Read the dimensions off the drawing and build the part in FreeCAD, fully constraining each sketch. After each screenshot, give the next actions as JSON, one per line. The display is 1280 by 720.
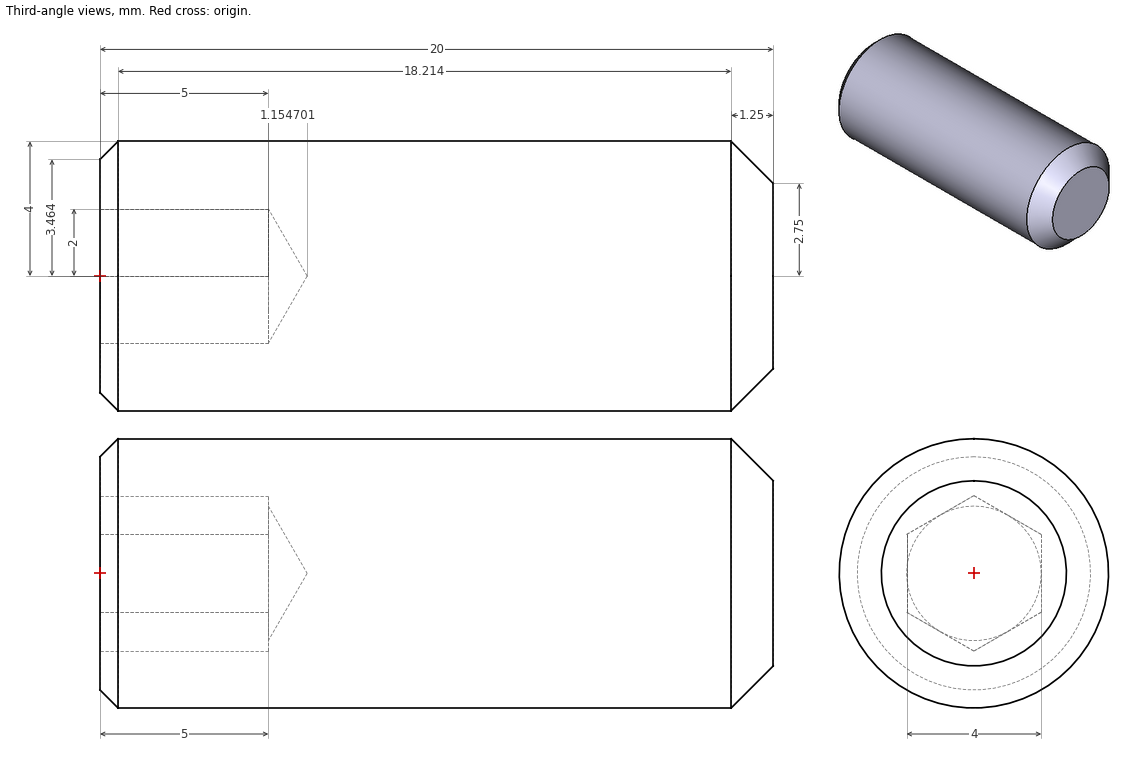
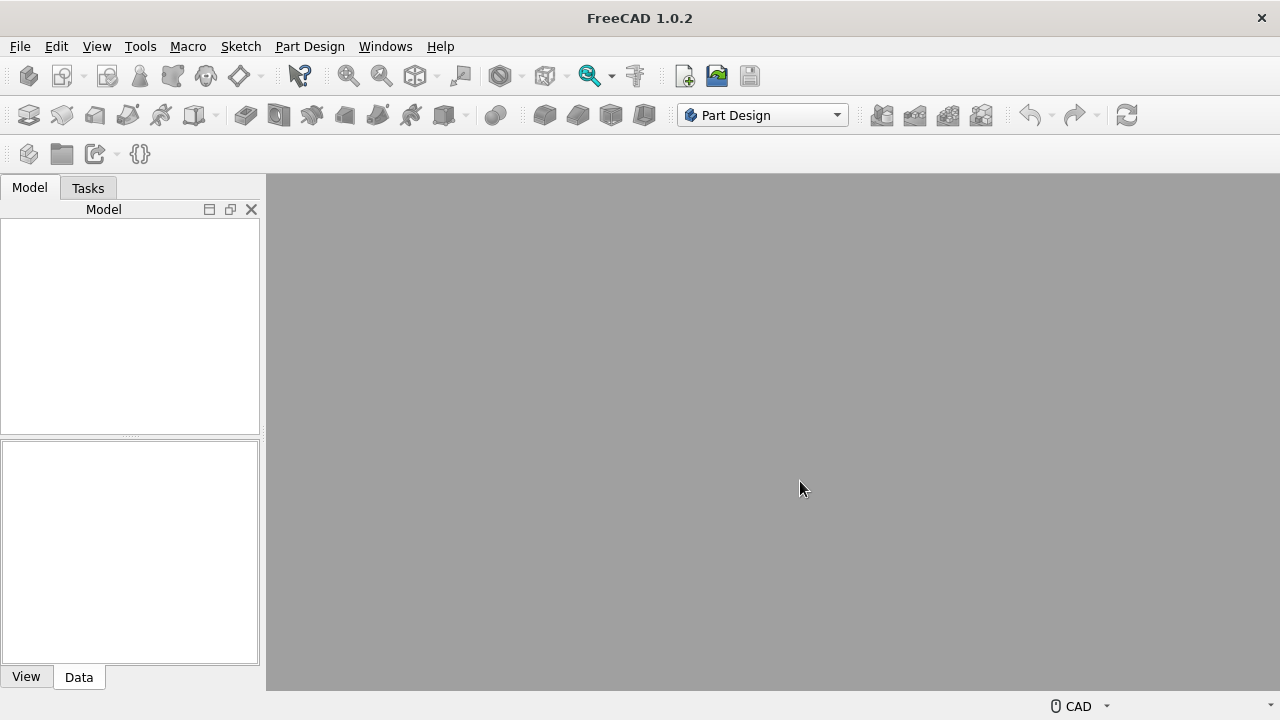
{"action": "left_click", "coordinate": [684, 76]}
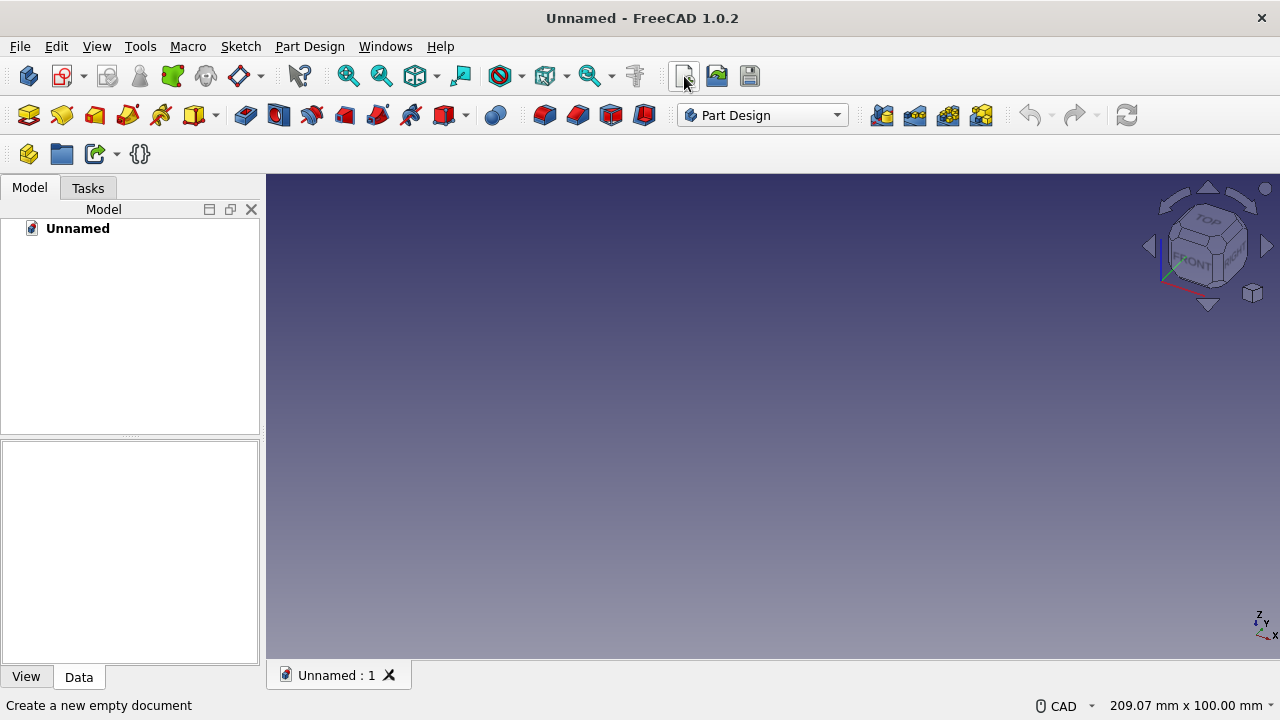
{"action": "left_click", "coordinate": [62, 76]}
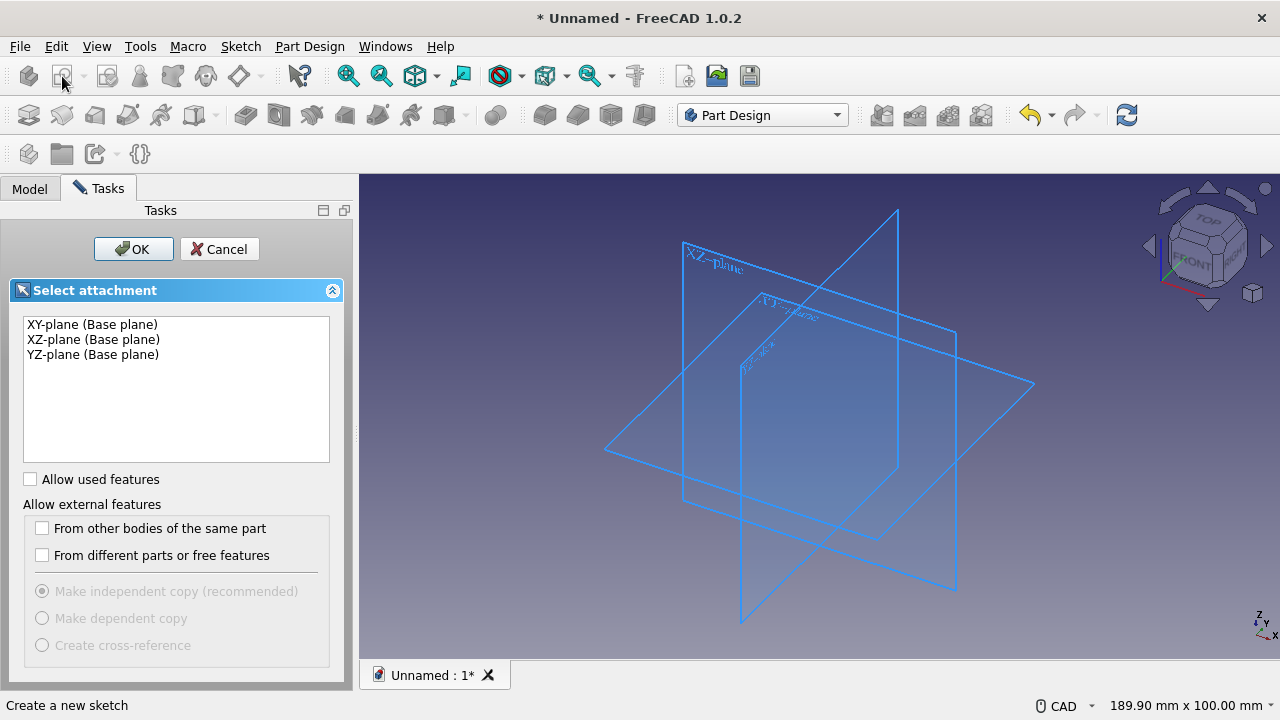
{"action": "left_click", "coordinate": [84, 324]}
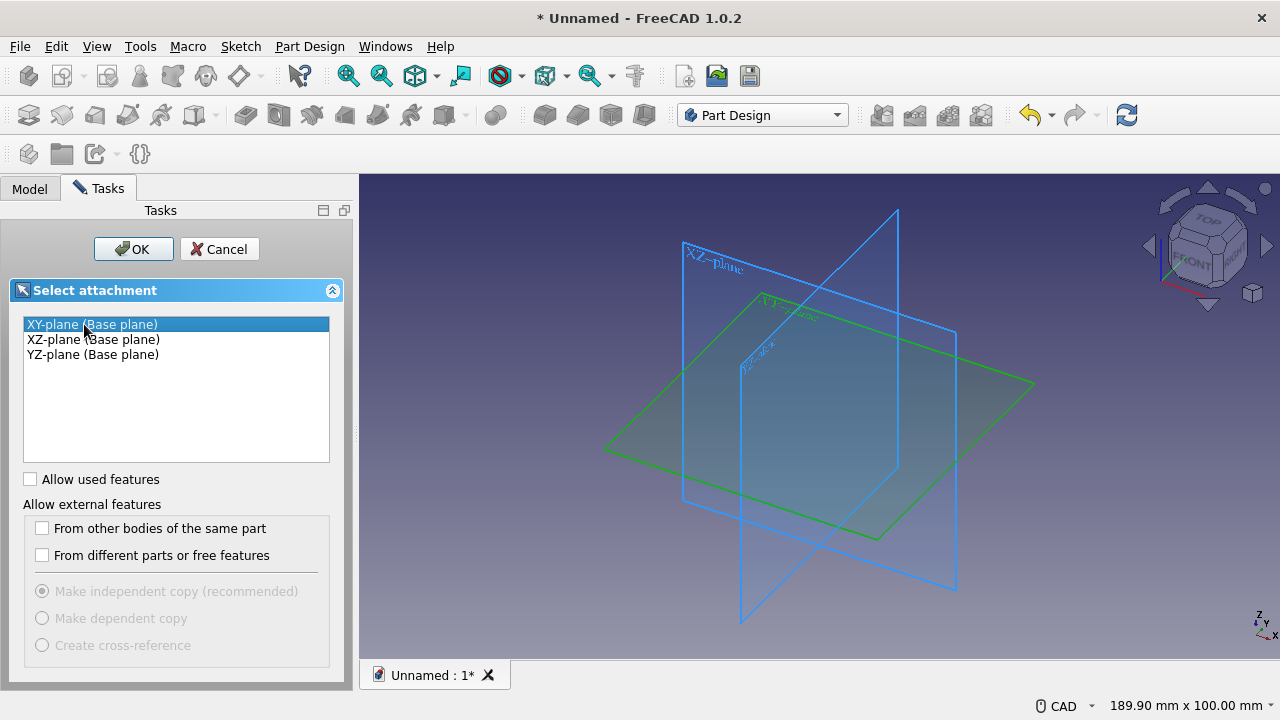
{"action": "left_click", "coordinate": [134, 249]}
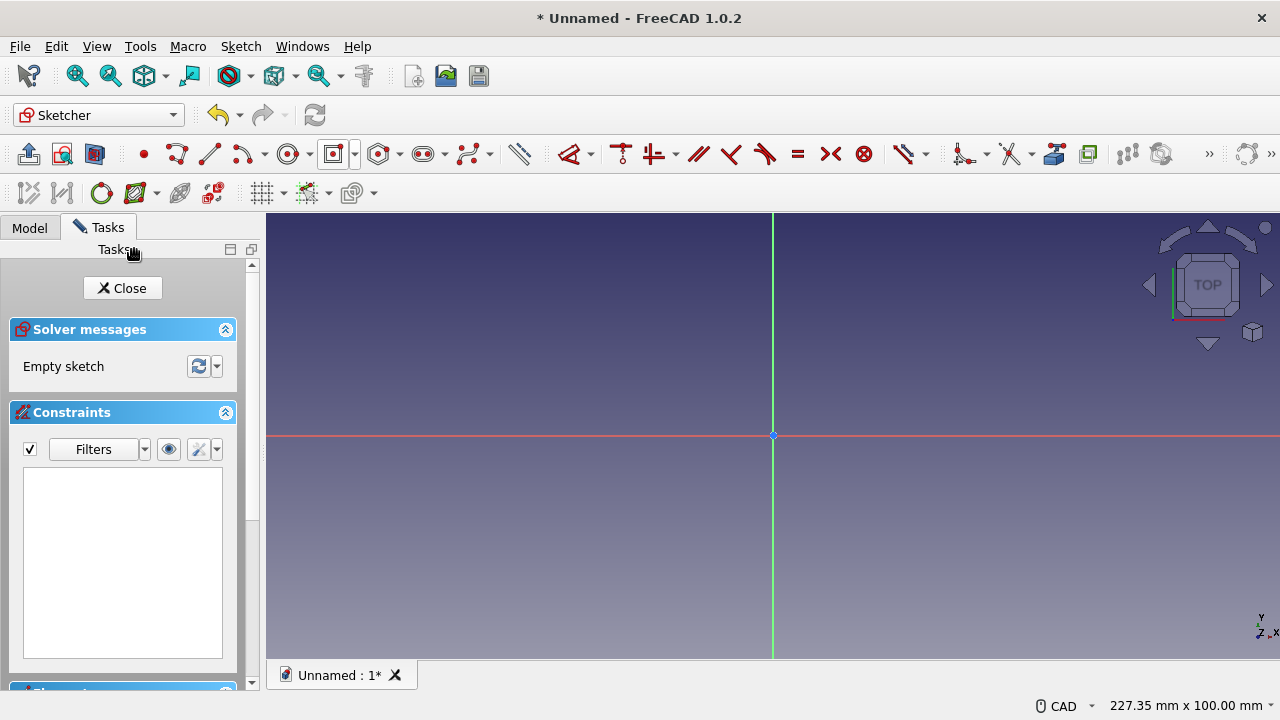
{"action": "scroll", "coordinate": [840, 425], "scroll_direction": "up", "scroll_amount": 9}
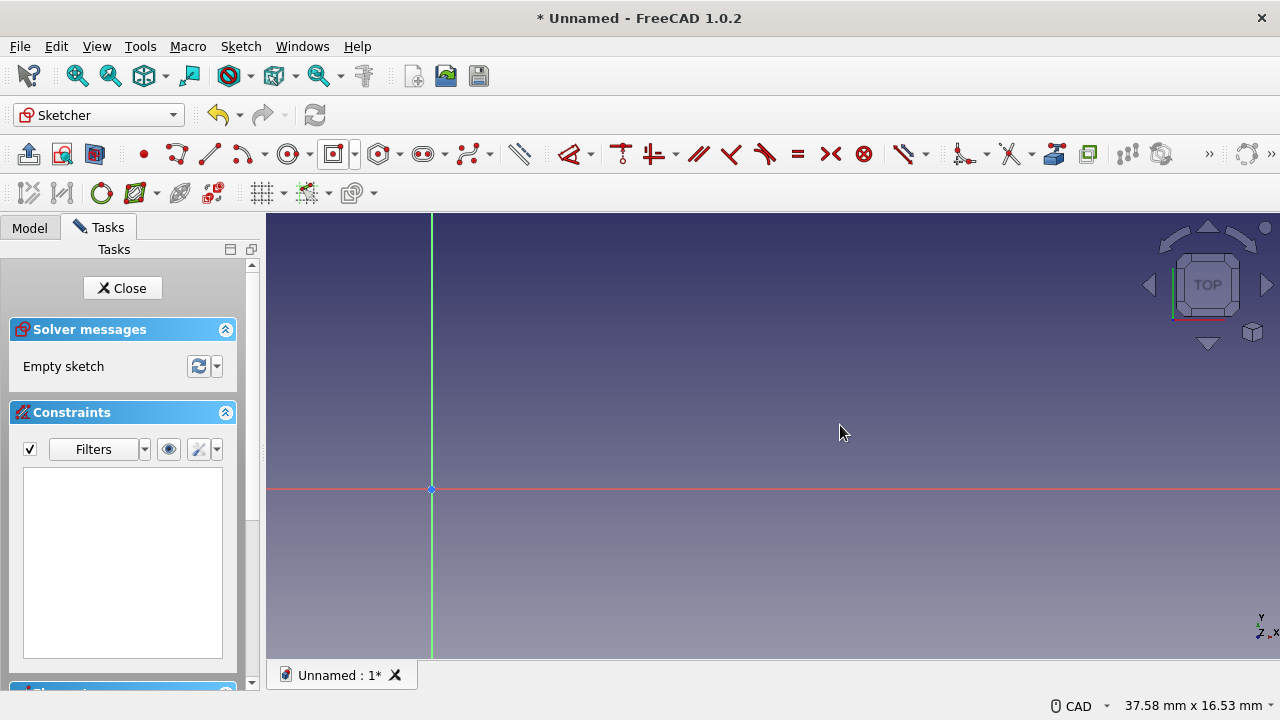
{"action": "key", "text": "g m"}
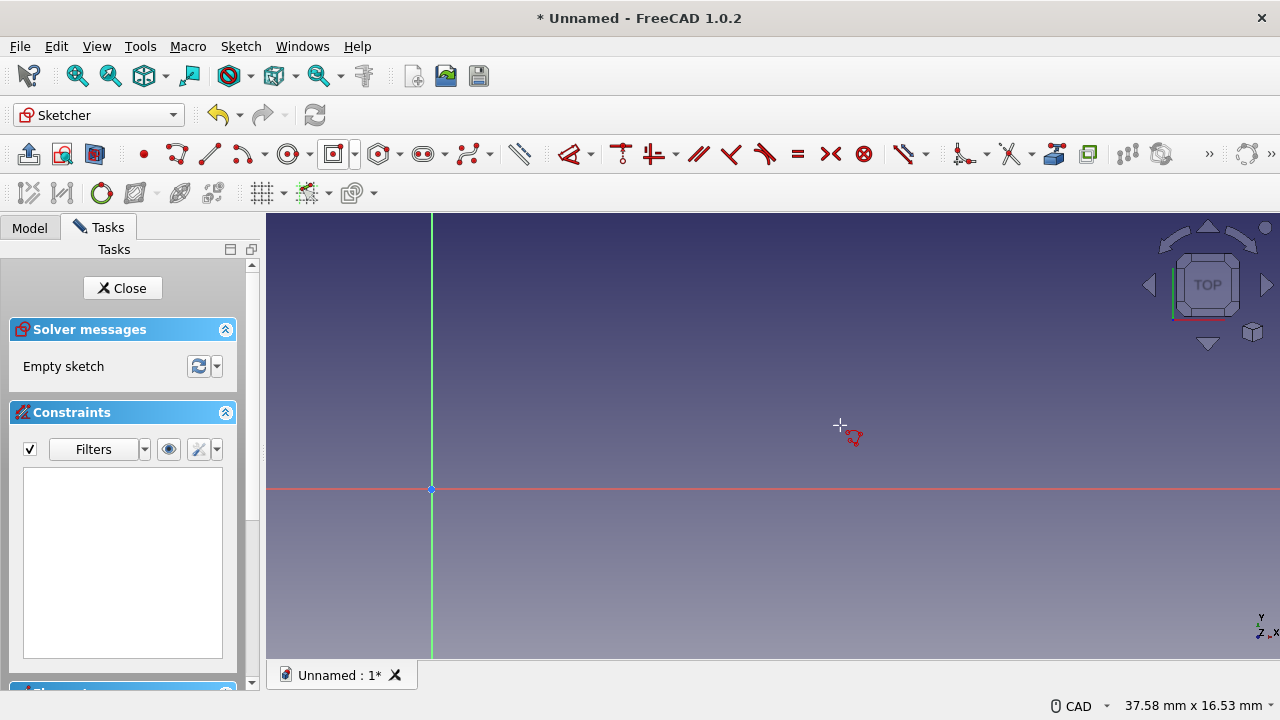
{"action": "left_click", "coordinate": [432, 489]}
{"action": "left_click", "coordinate": [971, 480]}
{"action": "left_click", "coordinate": [971, 415]}
{"action": "left_click", "coordinate": [938, 381]}
{"action": "left_click", "coordinate": [446, 381]}
{"action": "left_click", "coordinate": [441, 396]}
{"action": "left_click", "coordinate": [432, 489]}
{"action": "key", "text": "Escape"}
{"action": "key", "text": "Escape"}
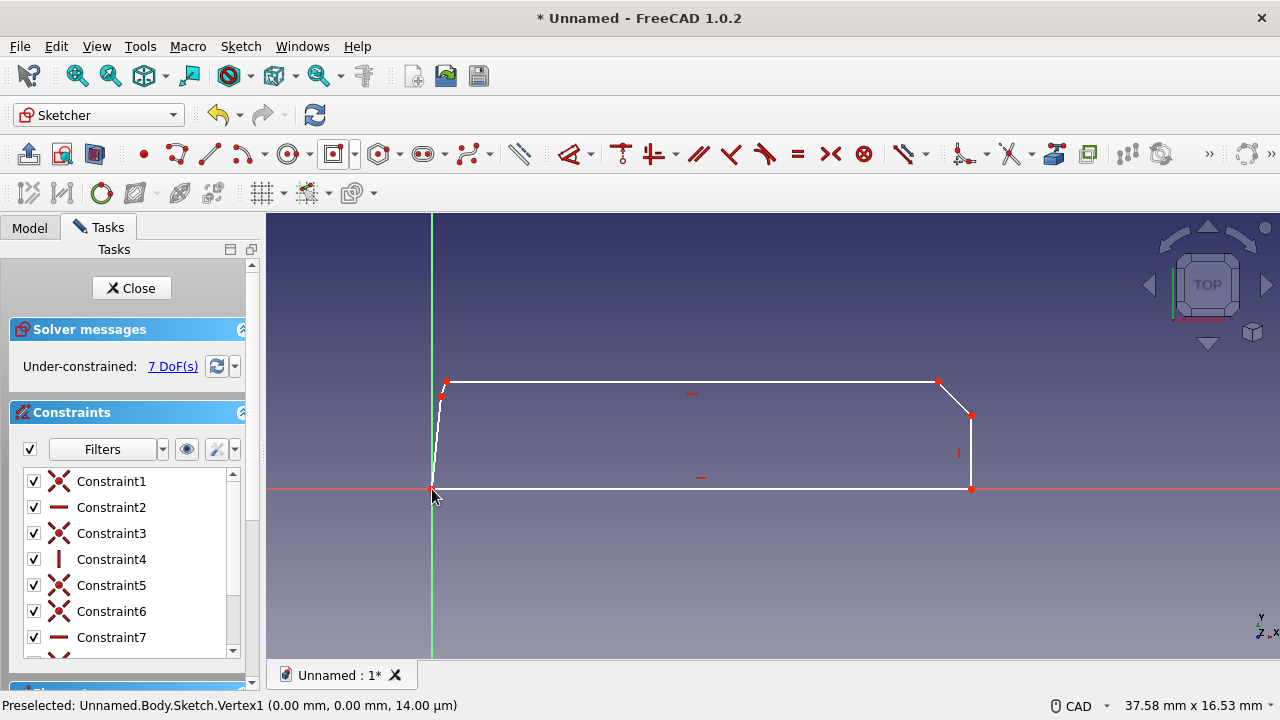
{"action": "left_click", "coordinate": [435, 461]}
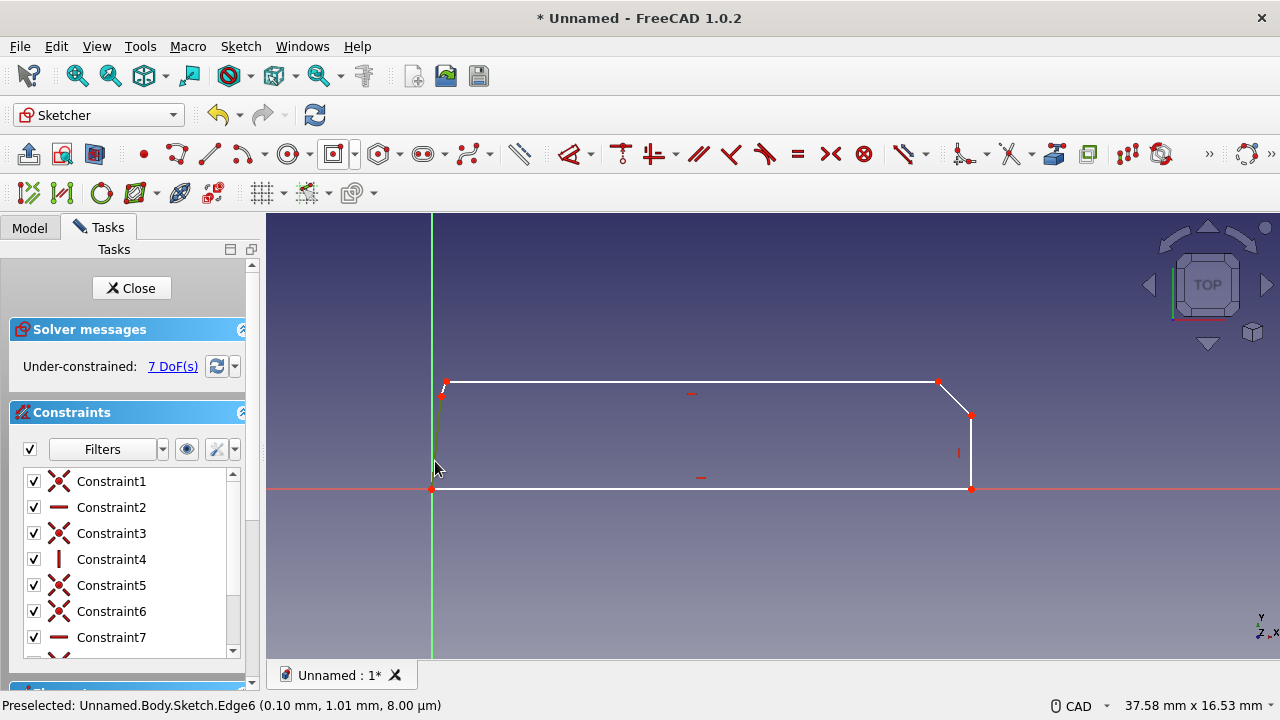
{"action": "left_click", "coordinate": [676, 154]}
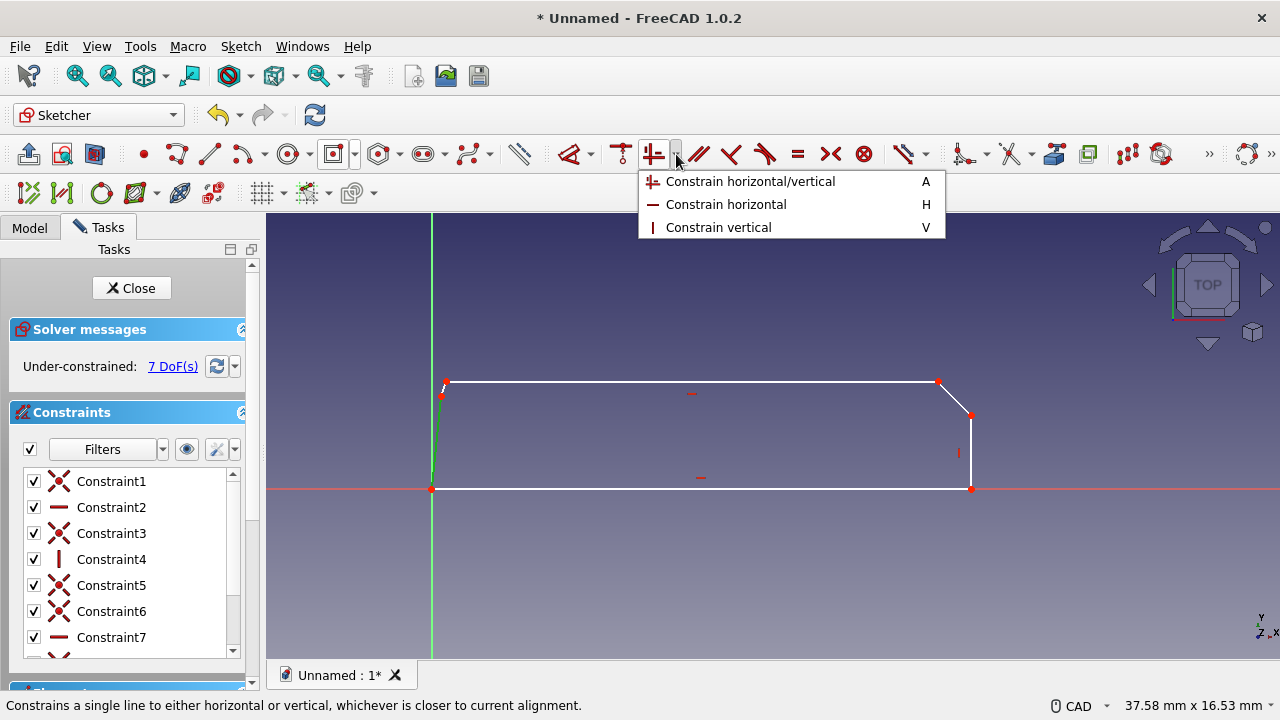
{"action": "left_click", "coordinate": [792, 228]}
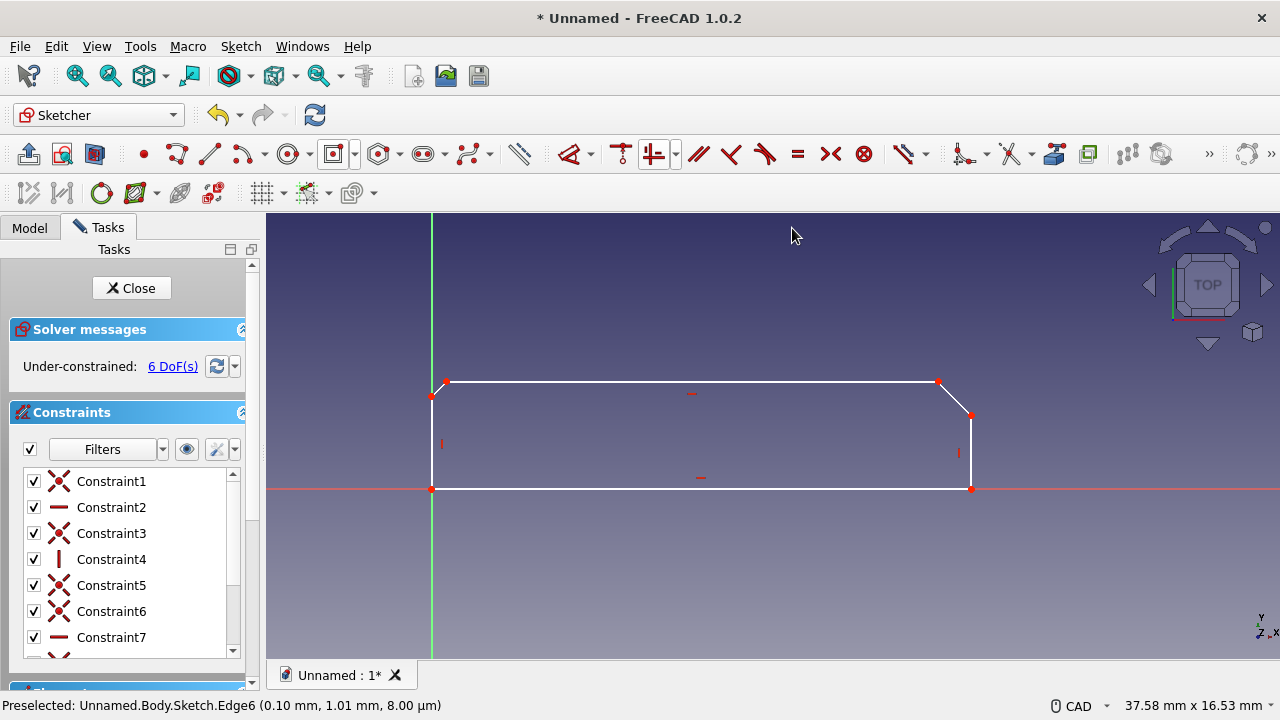
{"action": "left_click", "coordinate": [568, 154]}